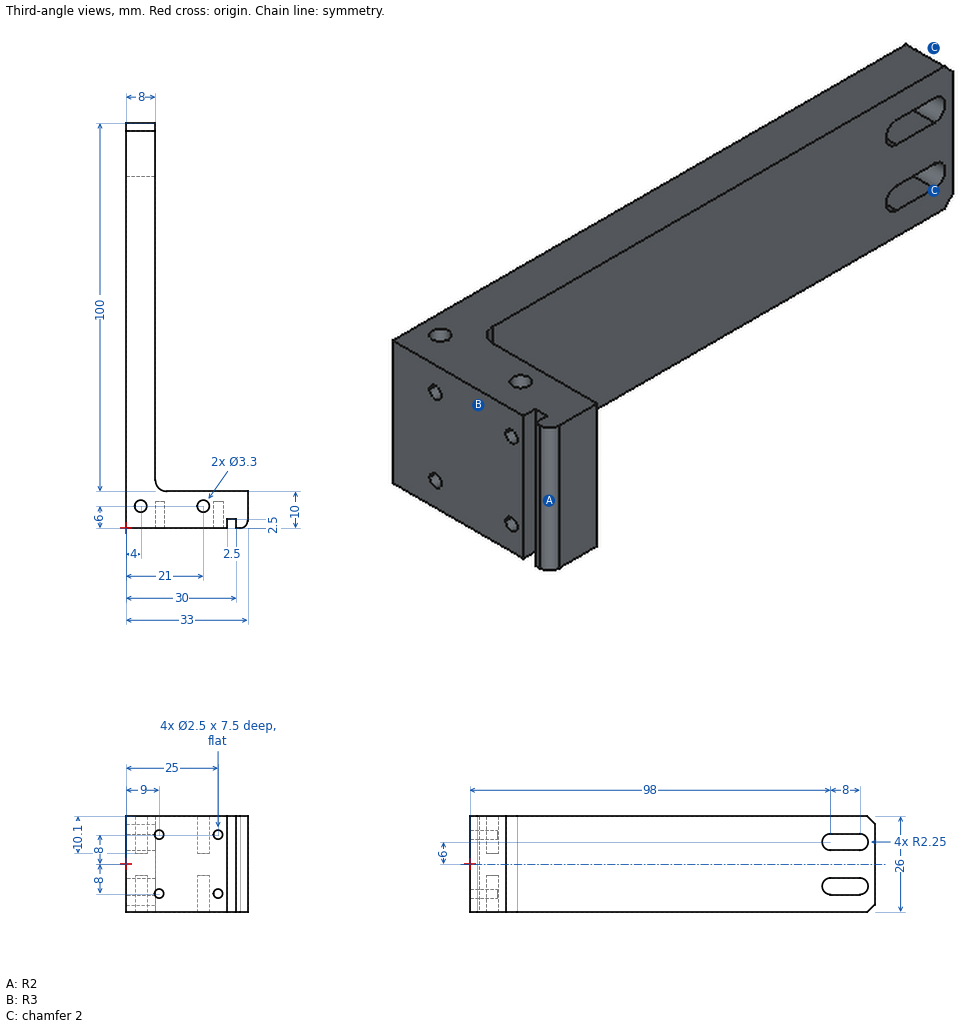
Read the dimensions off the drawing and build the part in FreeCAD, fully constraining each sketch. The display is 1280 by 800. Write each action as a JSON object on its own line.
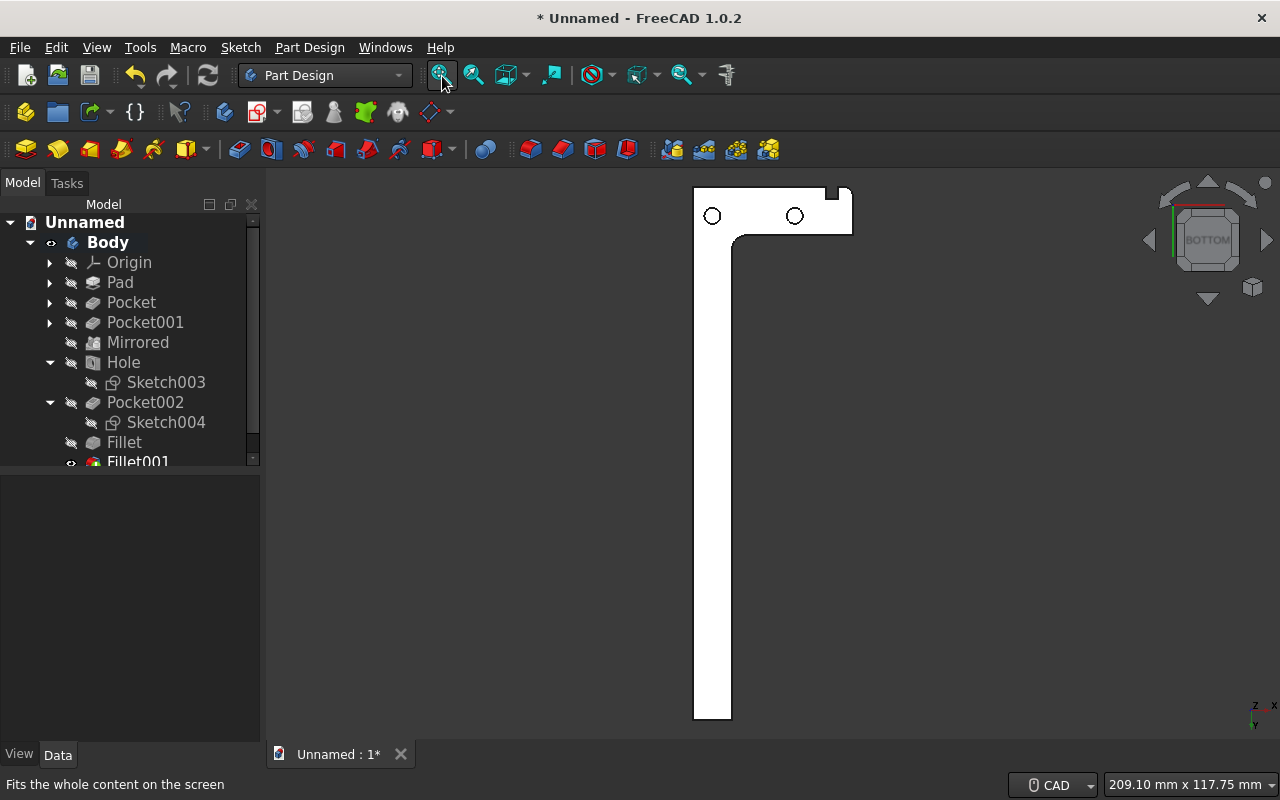
{"action": "key", "text": "4"}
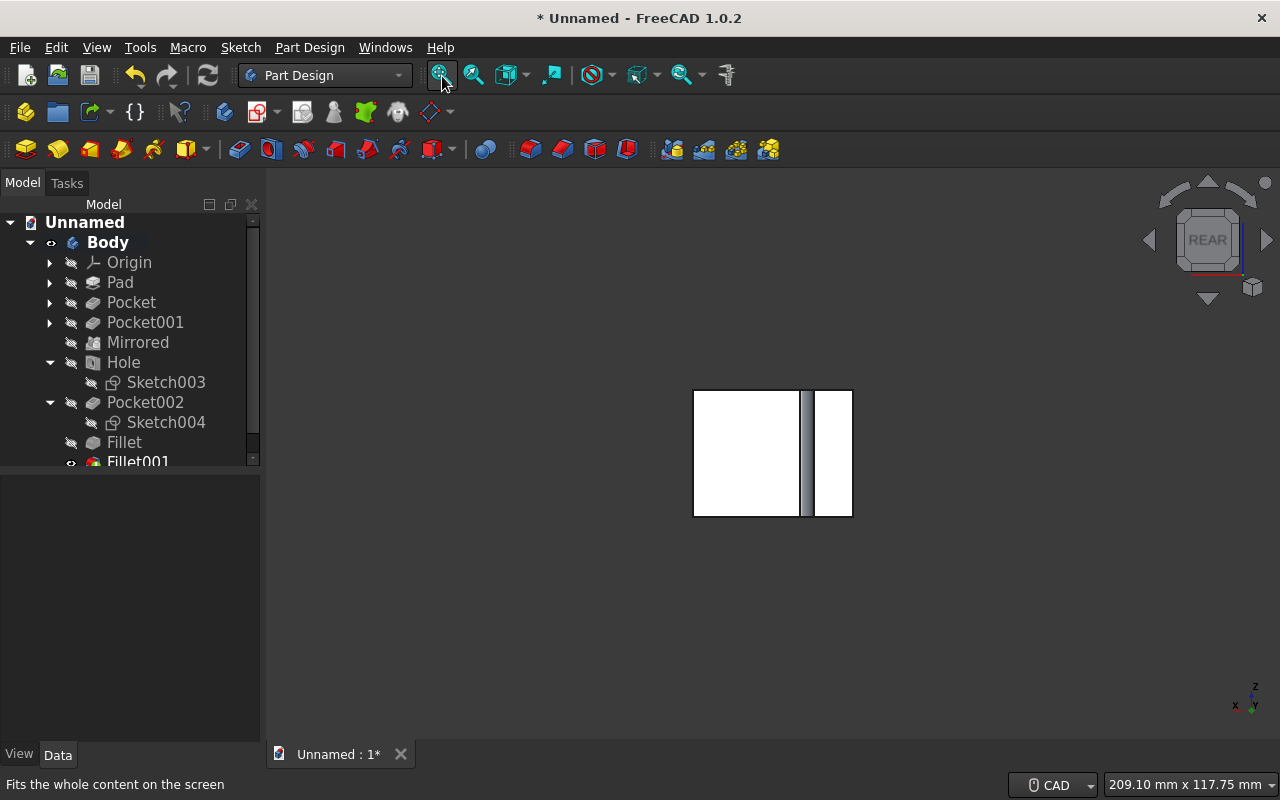
{"action": "left_click", "coordinate": [442, 76]}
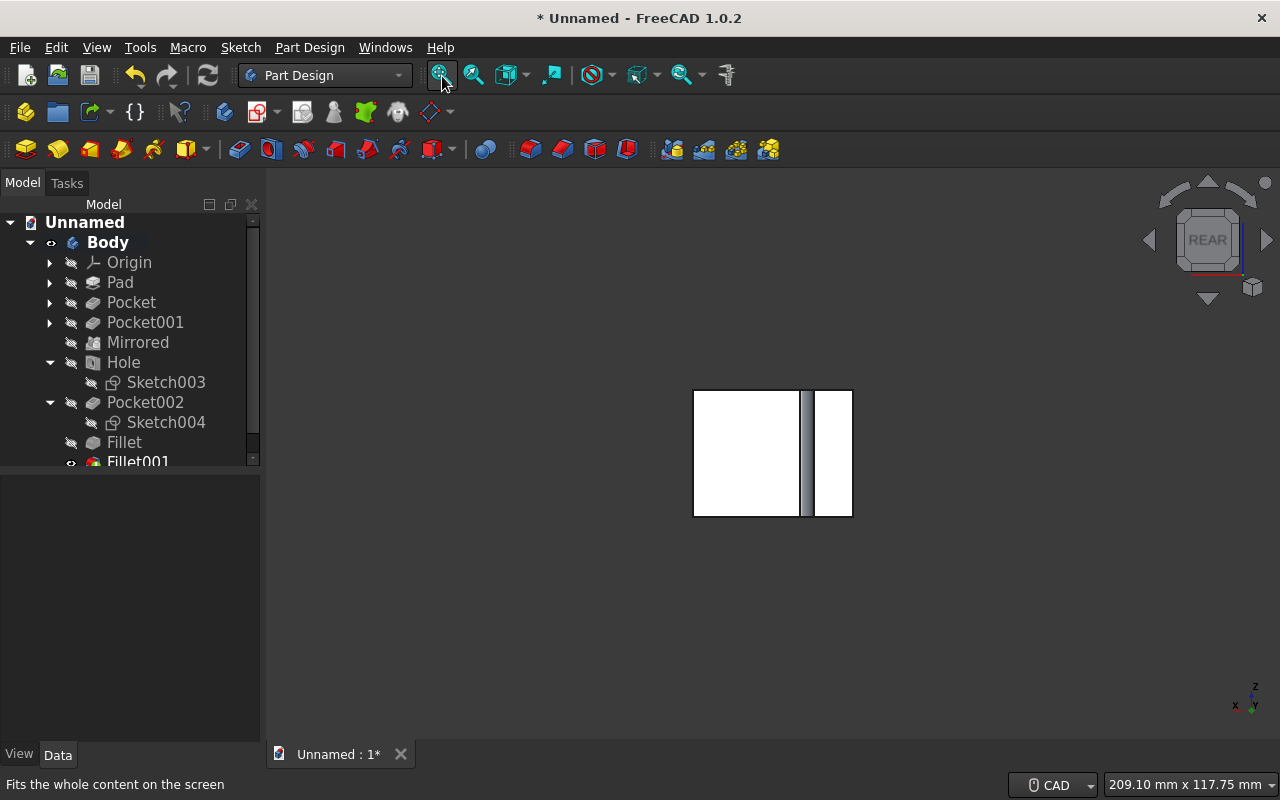
{"action": "left_click", "coordinate": [834, 389]}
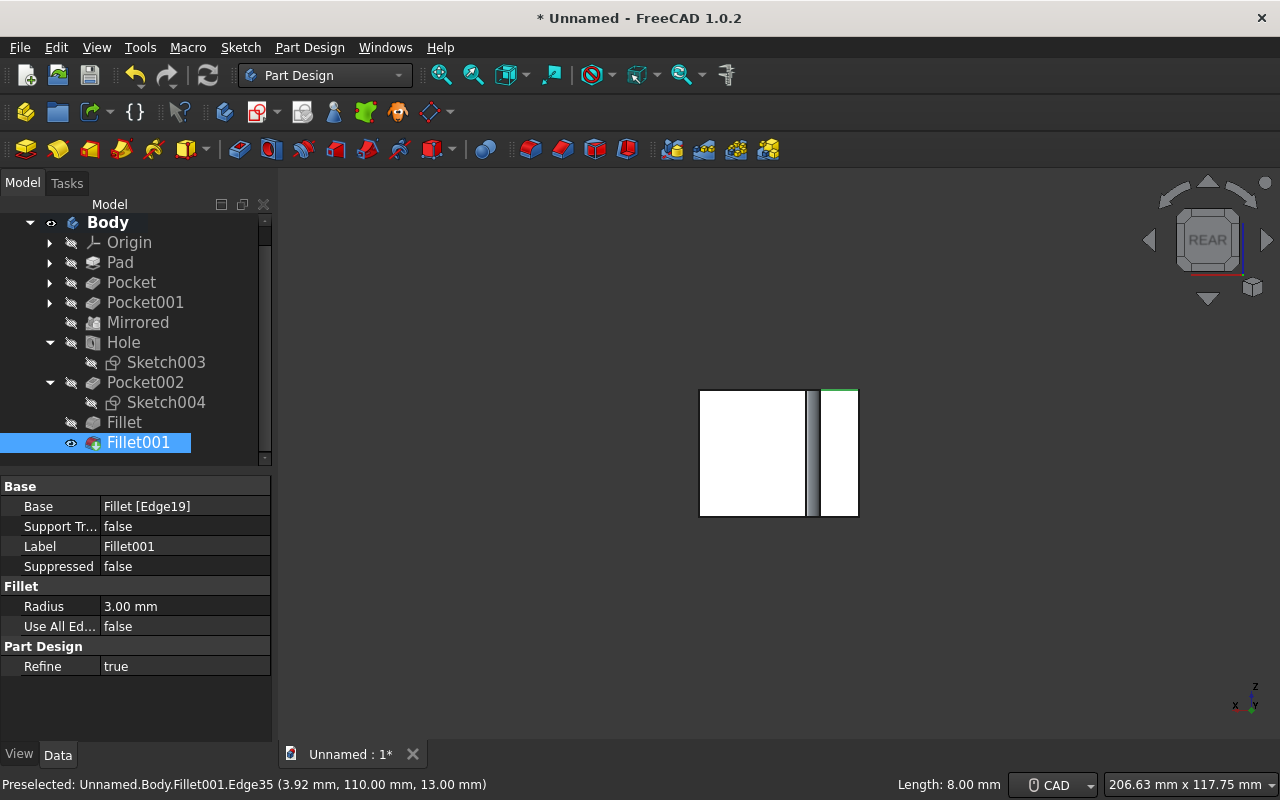
{"action": "left_click", "coordinate": [840, 516], "text": "ctrl"}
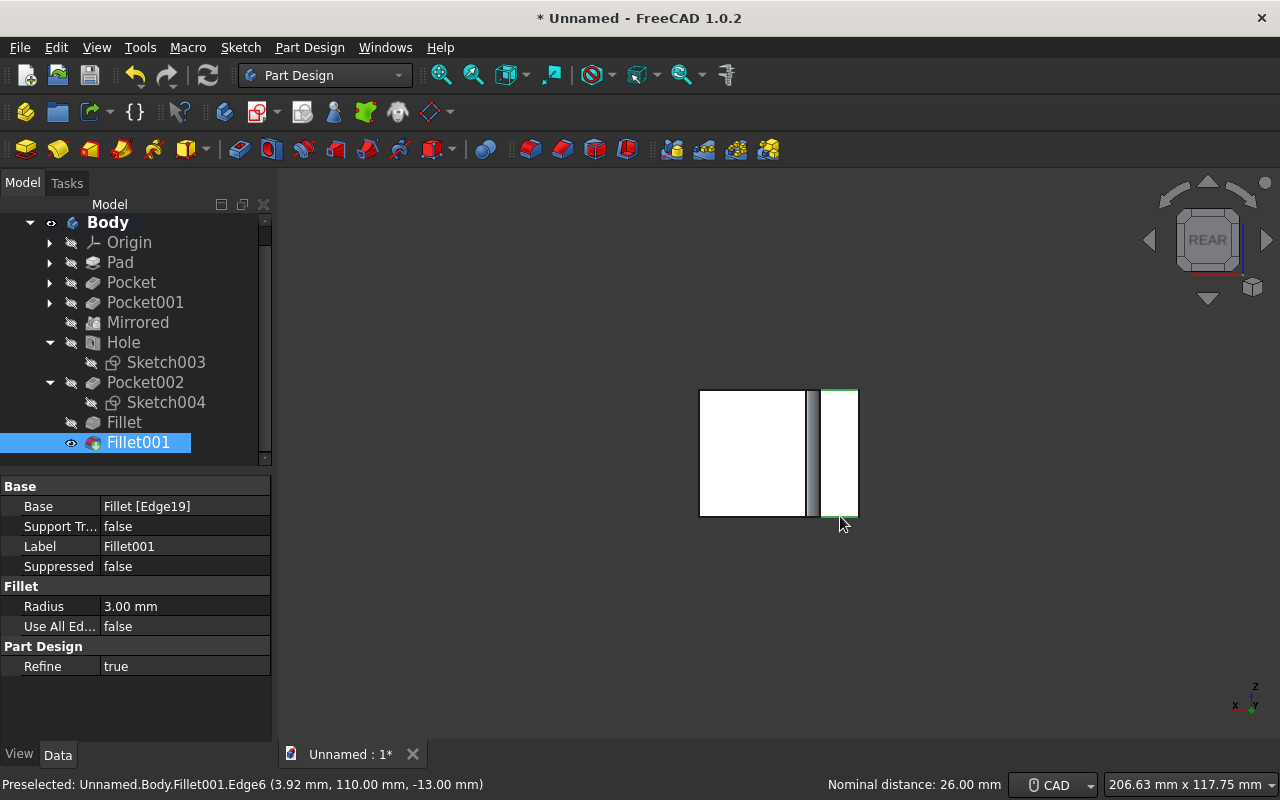
{"action": "left_click", "coordinate": [564, 150]}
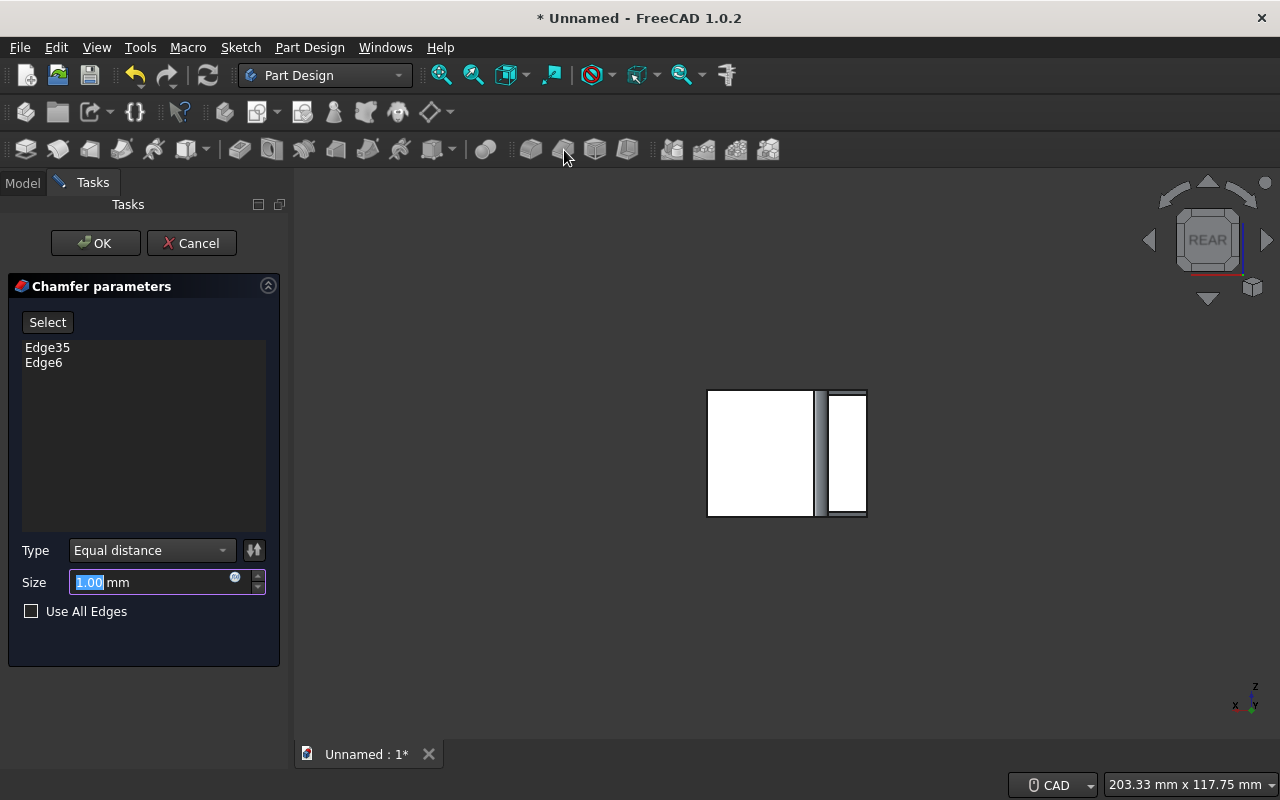
{"action": "type", "text": "2"}
{"action": "key", "text": "Tab"}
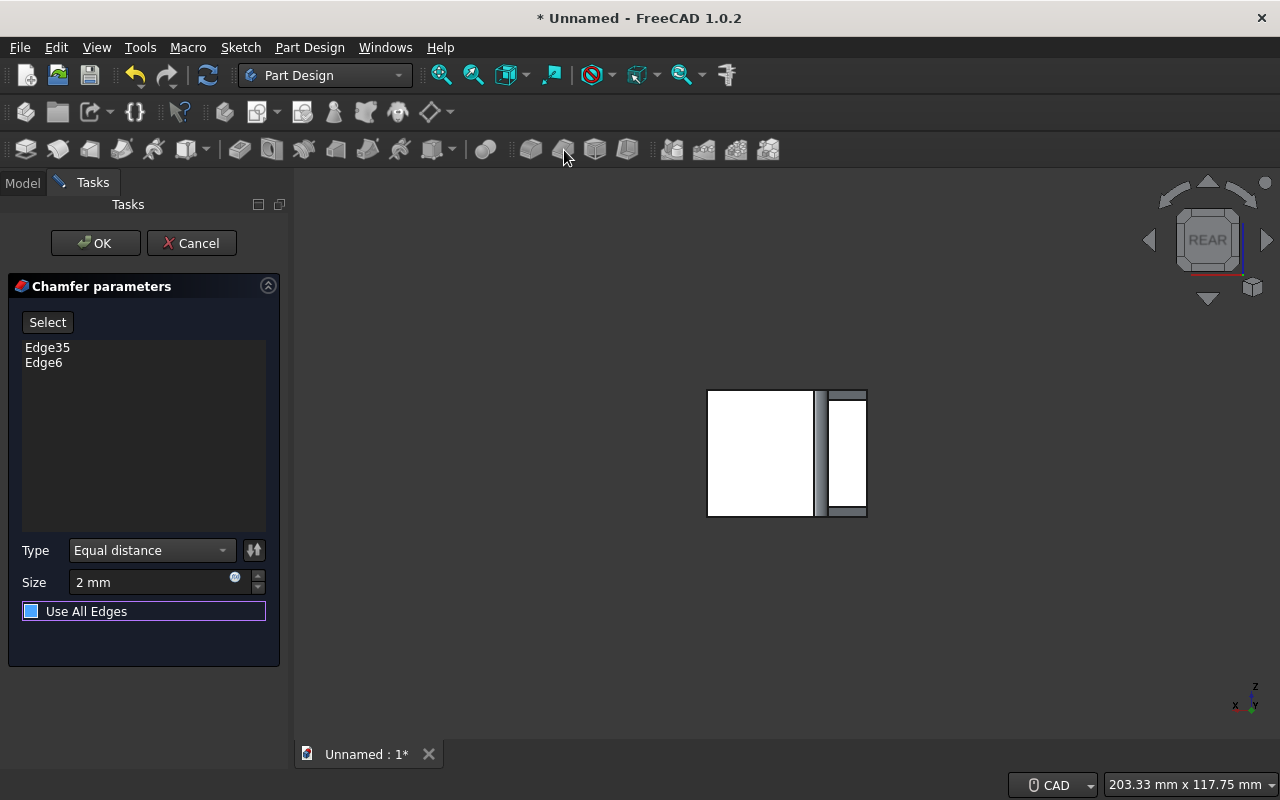
{"action": "left_click", "coordinate": [96, 243]}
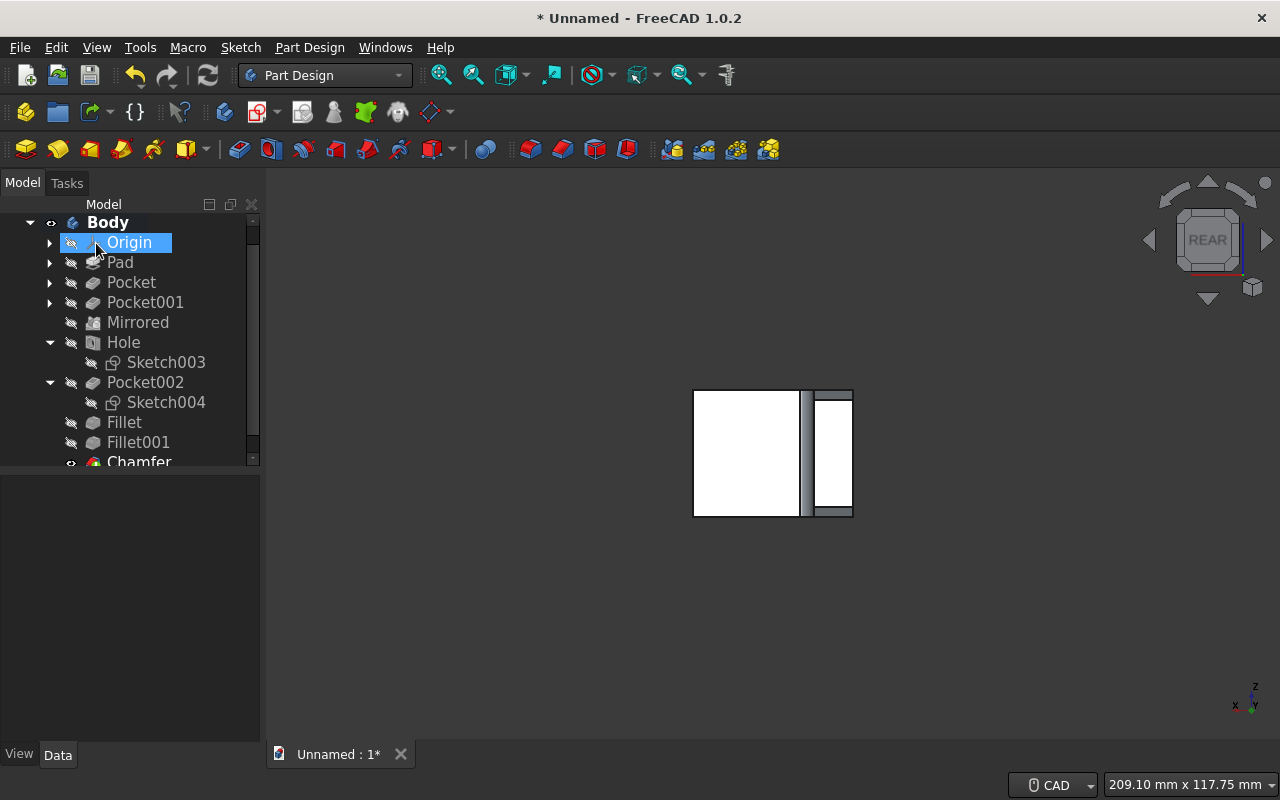
{"action": "key", "text": "0"}